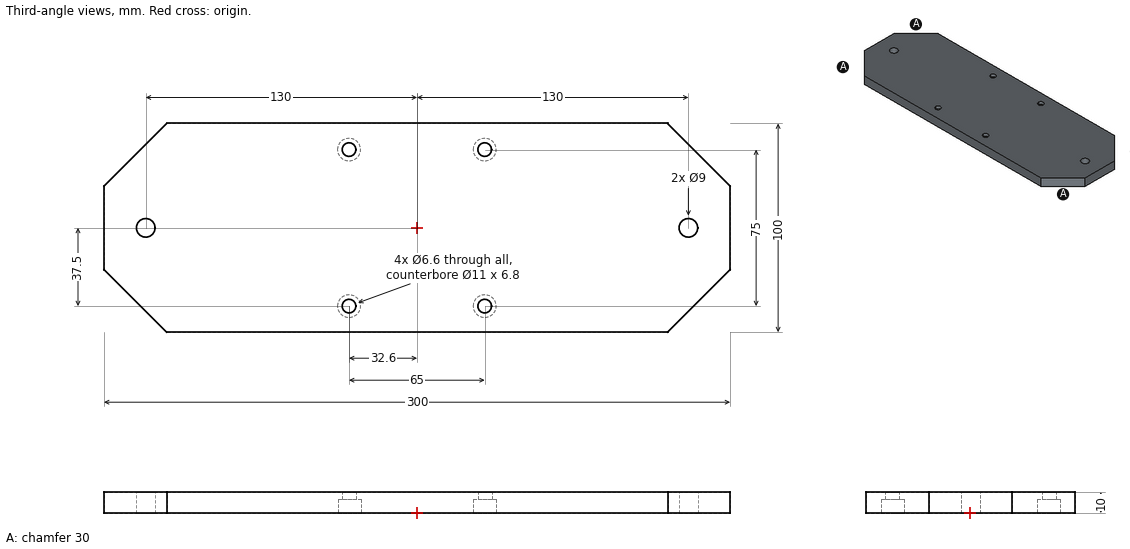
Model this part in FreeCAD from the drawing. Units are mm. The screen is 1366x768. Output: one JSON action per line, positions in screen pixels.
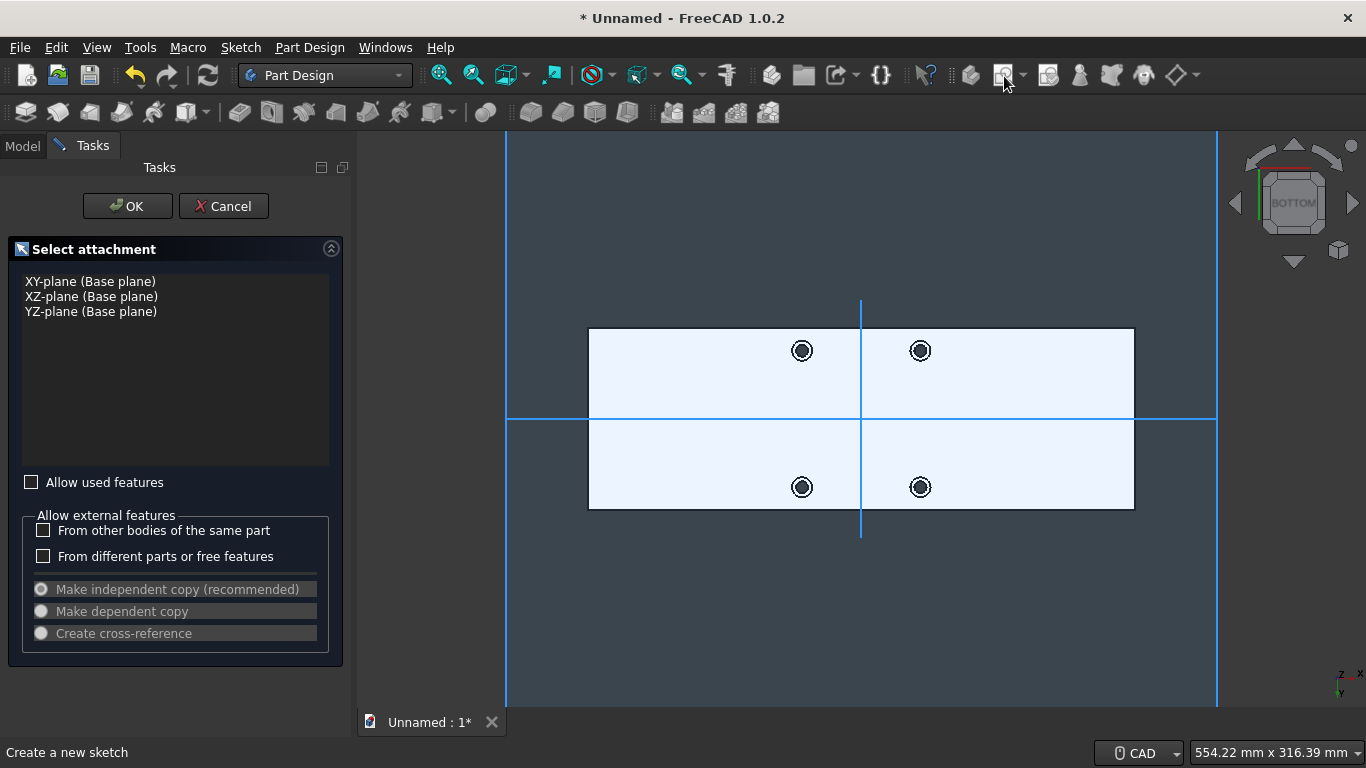
{"action": "left_click", "coordinate": [82, 282]}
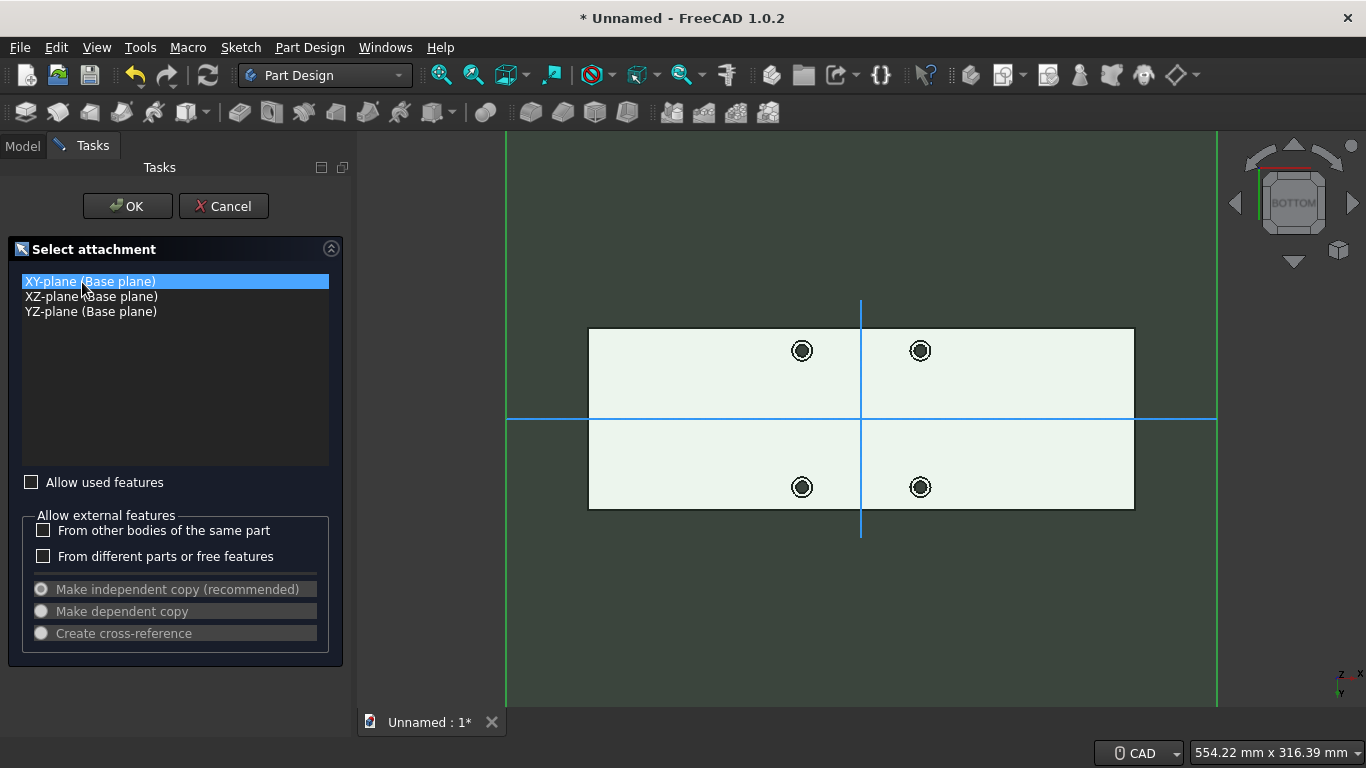
{"action": "left_click", "coordinate": [128, 206]}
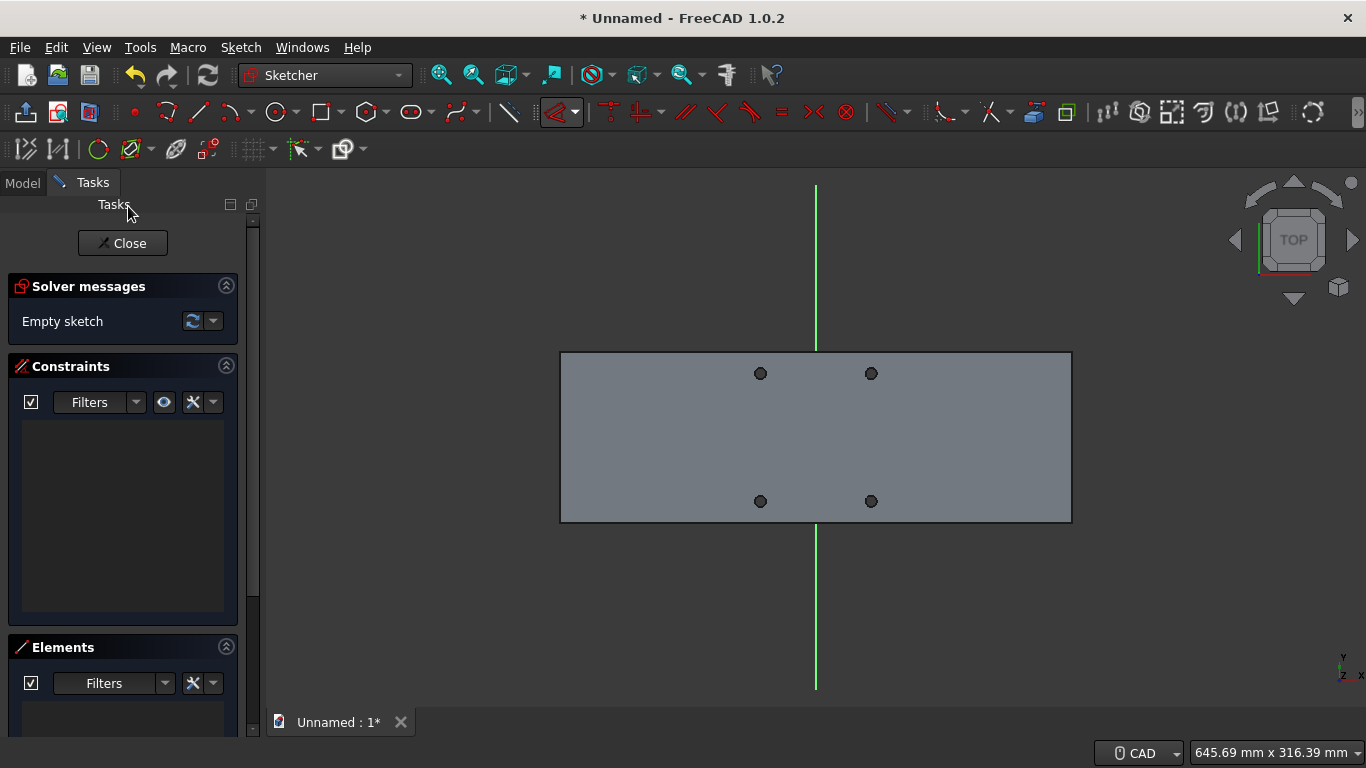
{"action": "left_click", "coordinate": [90, 112]}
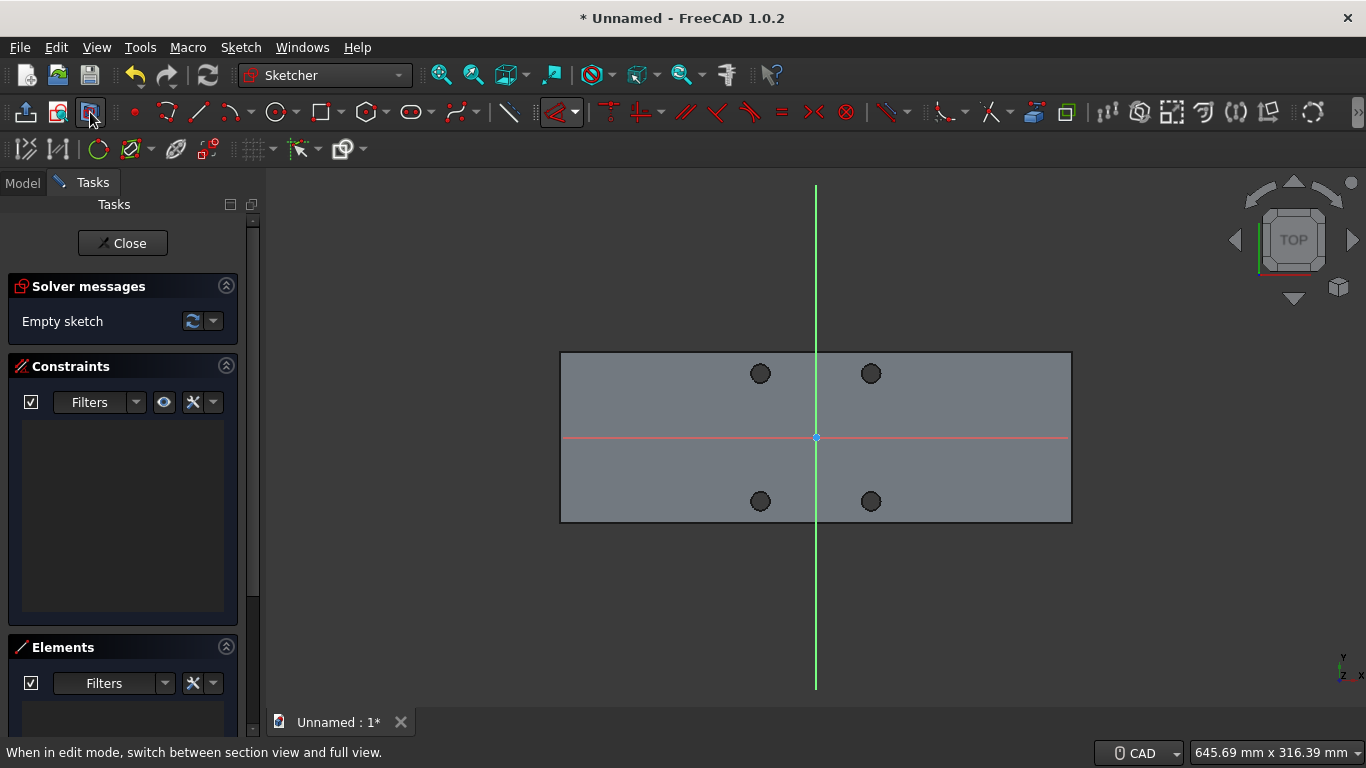
{"action": "scroll", "coordinate": [955, 437], "scroll_direction": "up", "scroll_amount": 2}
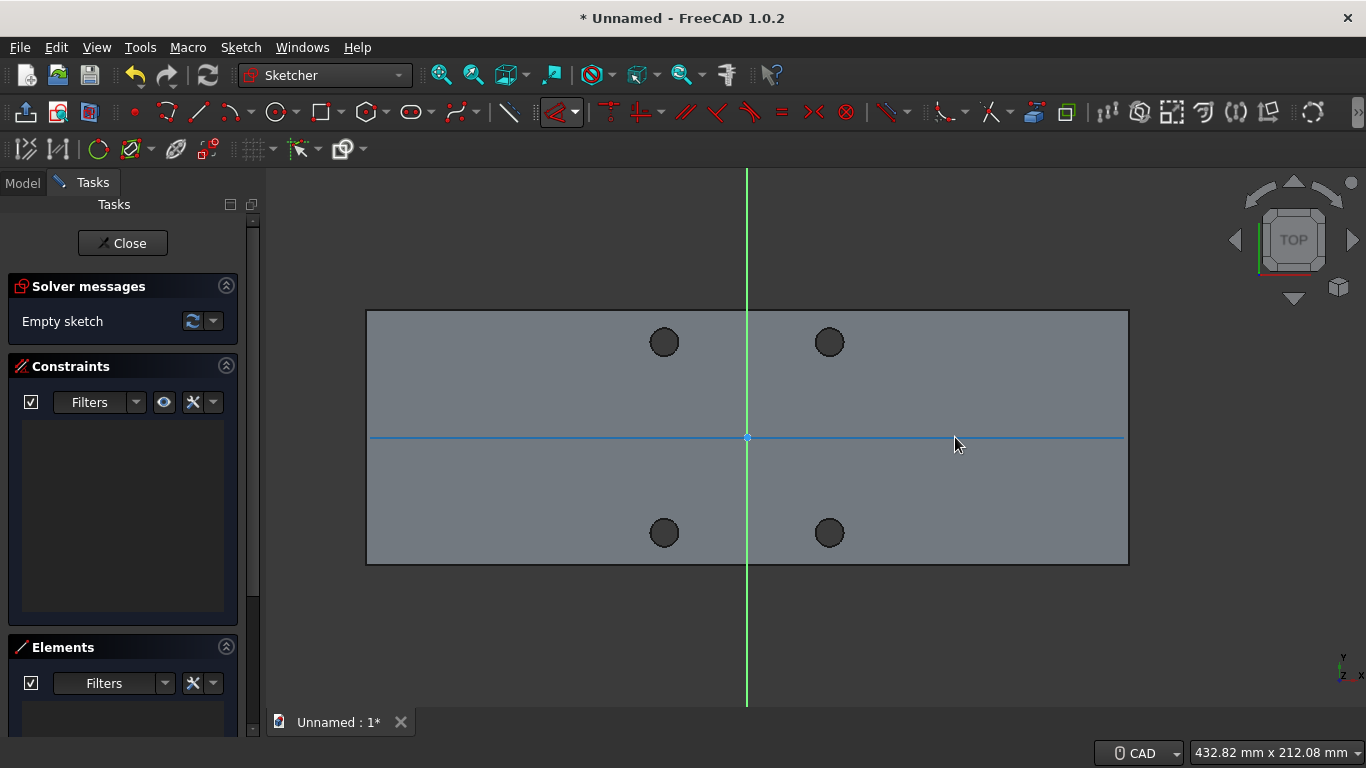
{"action": "left_click", "coordinate": [276, 112]}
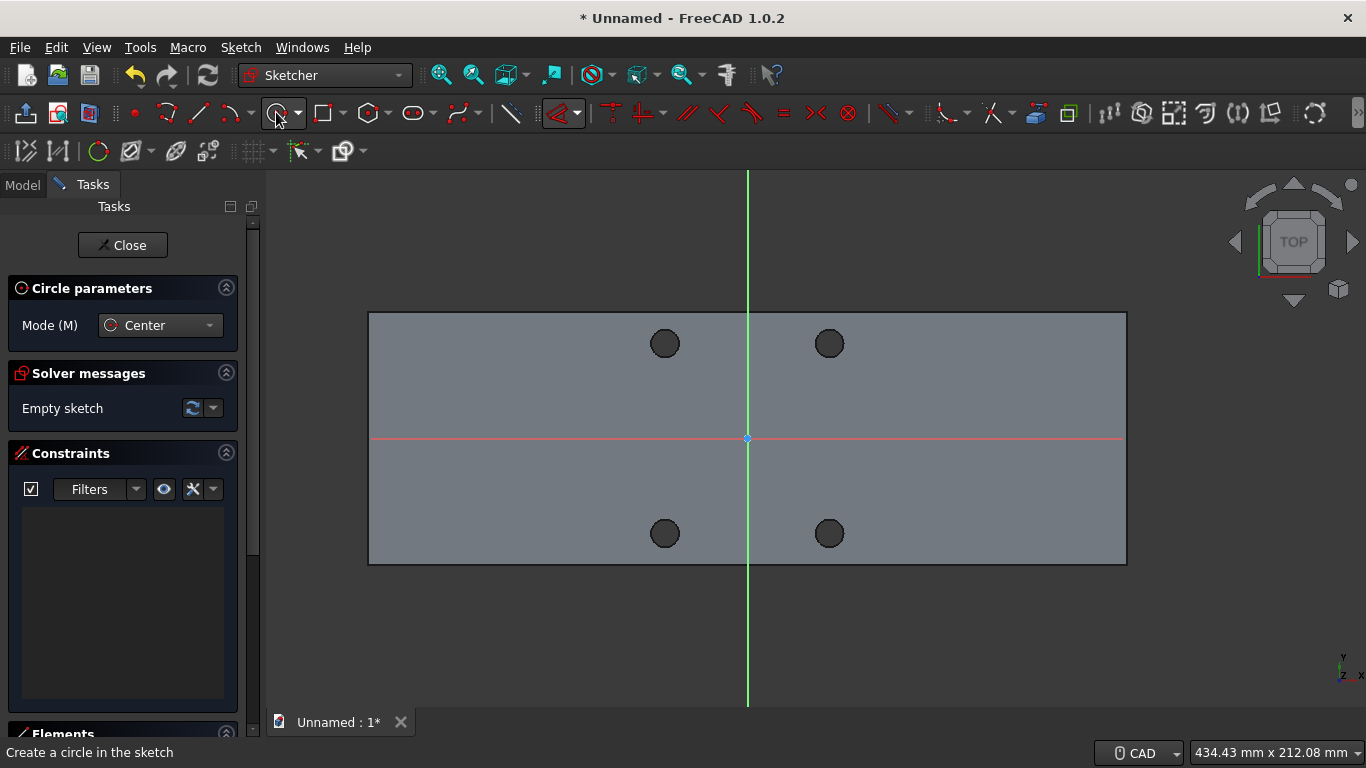
{"action": "scroll", "coordinate": [1077, 438], "scroll_direction": "up", "scroll_amount": 4}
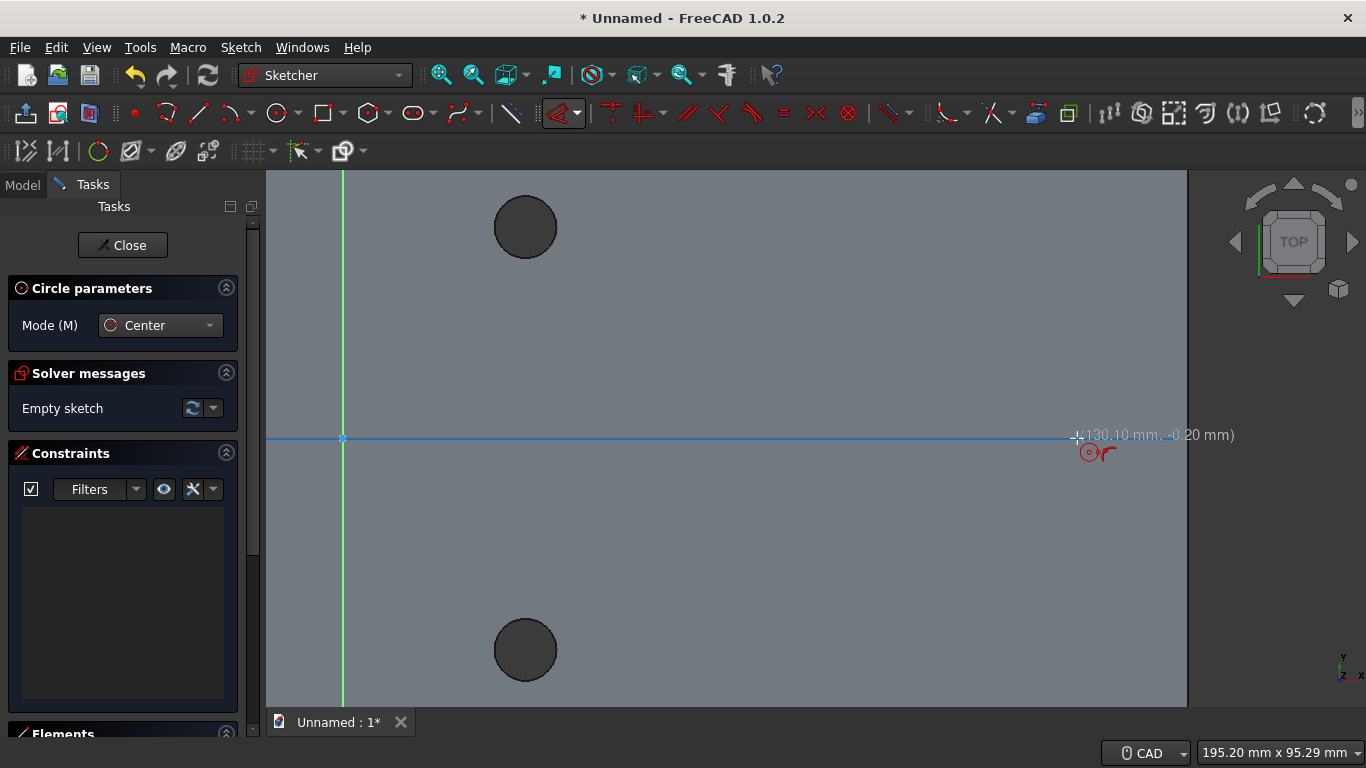
{"action": "left_click", "coordinate": [1076, 438]}
{"action": "mouse_move", "coordinate": [1093, 421]}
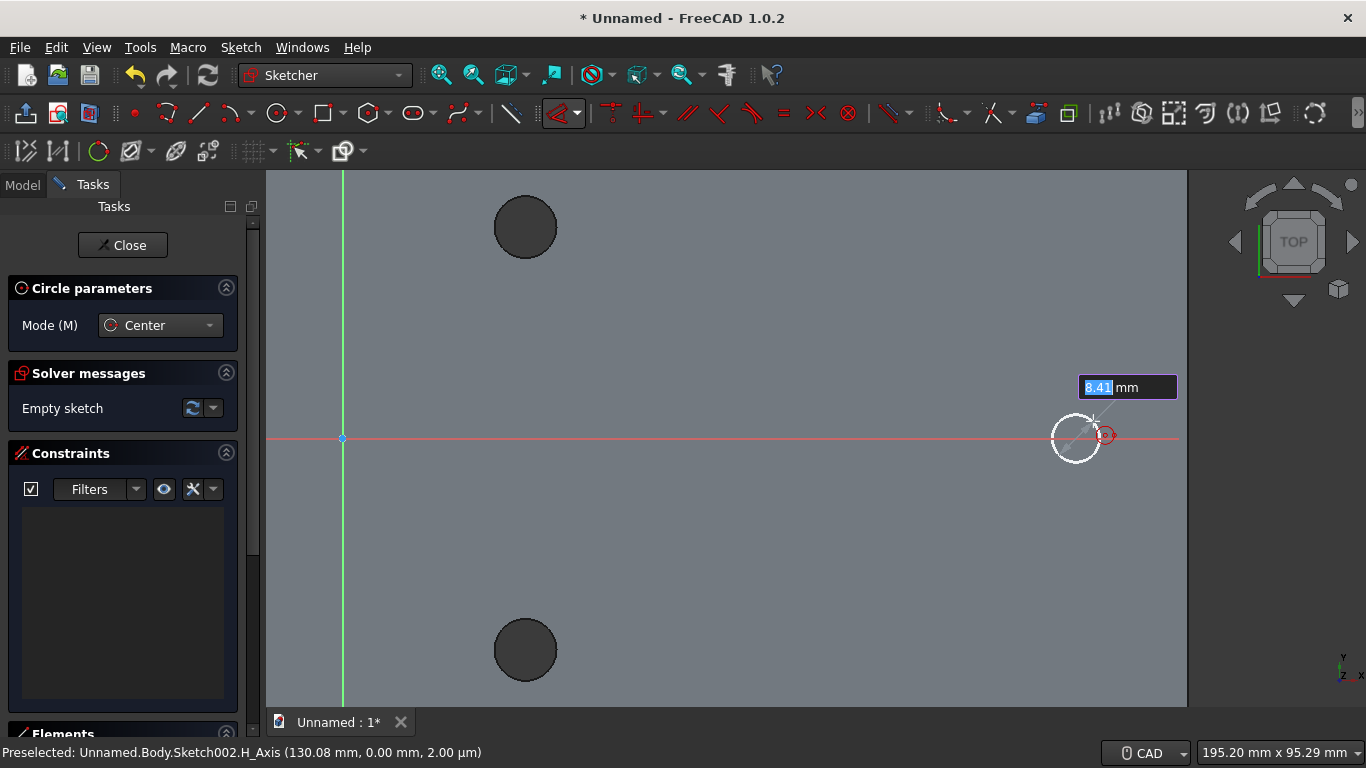
{"action": "type", "text": "9"}
{"action": "key", "text": "Return"}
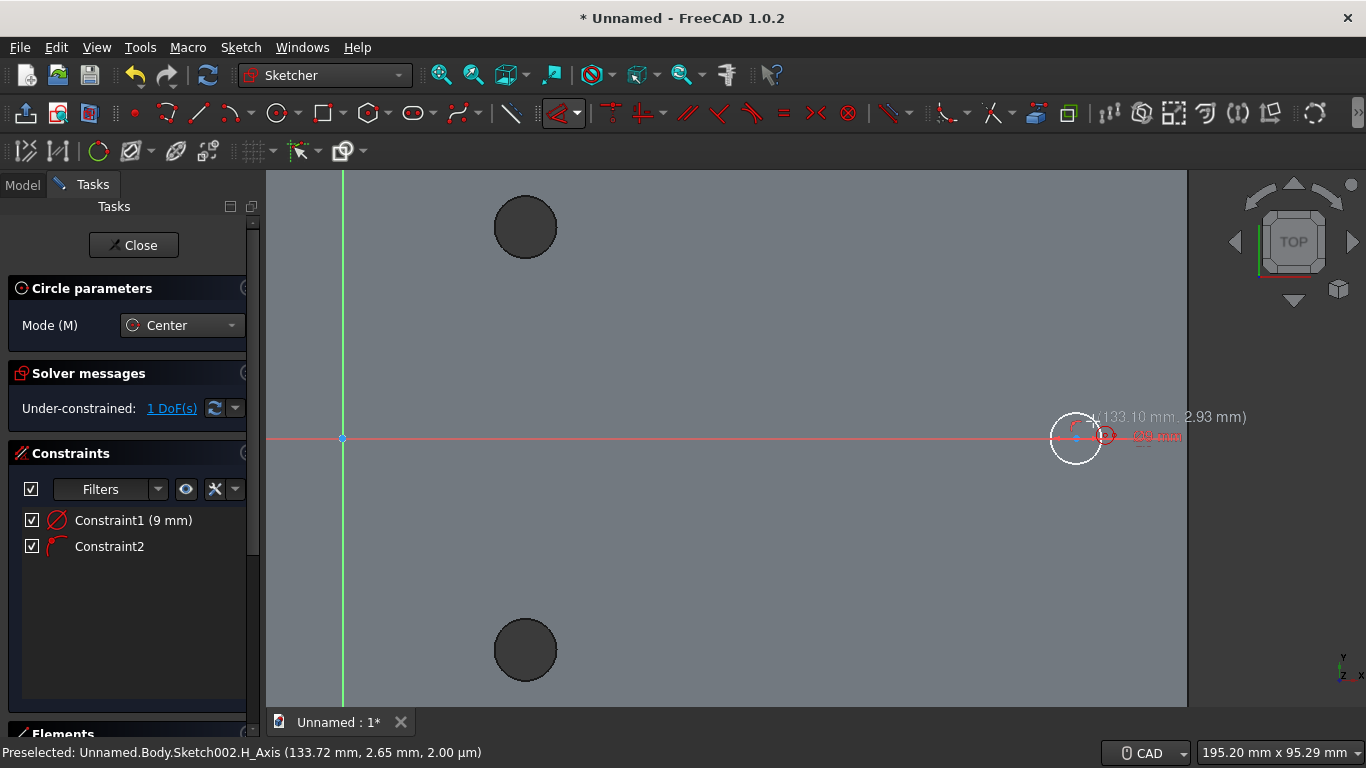
{"action": "scroll", "coordinate": [1078, 439], "scroll_direction": "down", "scroll_amount": 4}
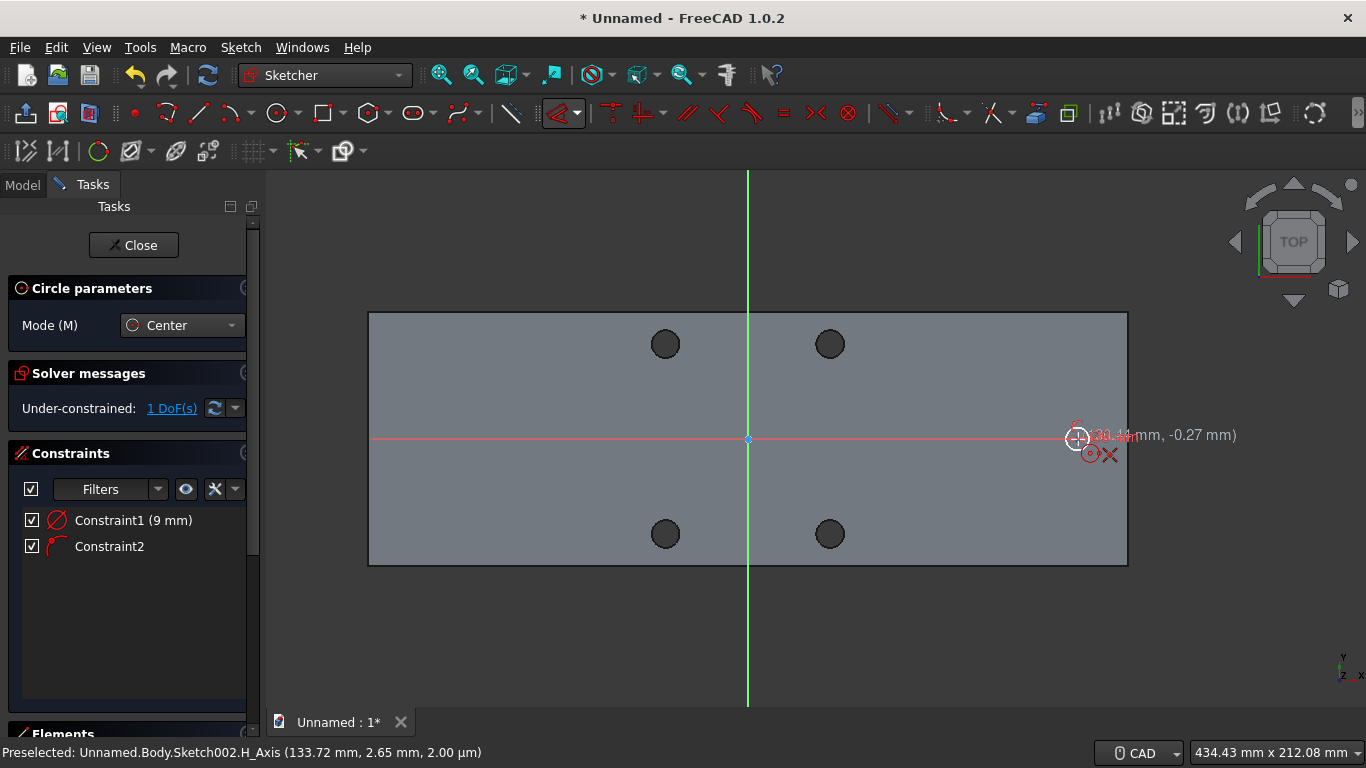
{"action": "scroll", "coordinate": [419, 439], "scroll_direction": "up", "scroll_amount": 4}